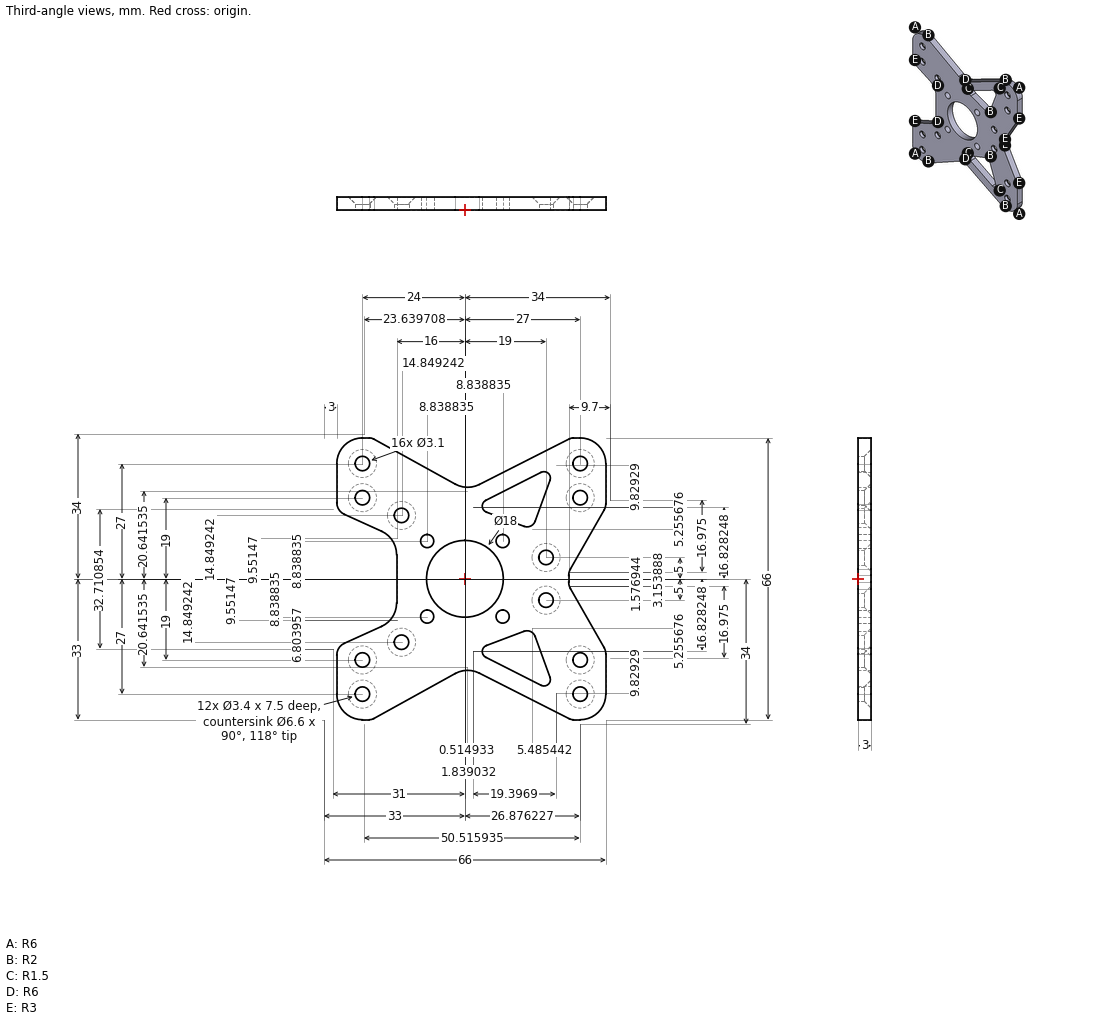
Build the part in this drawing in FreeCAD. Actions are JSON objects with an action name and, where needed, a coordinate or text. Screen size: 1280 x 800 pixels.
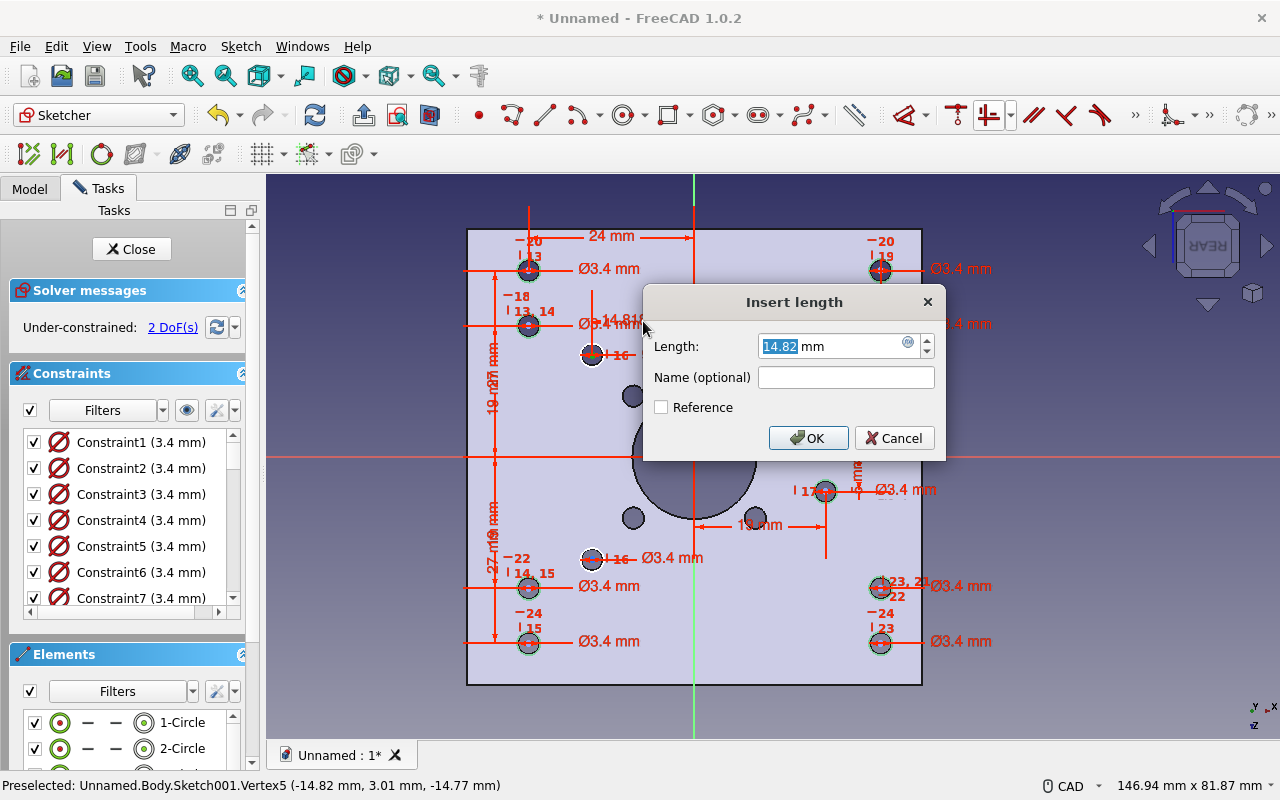
{"action": "type", "text": "14.849242"}
{"action": "key", "text": "Return"}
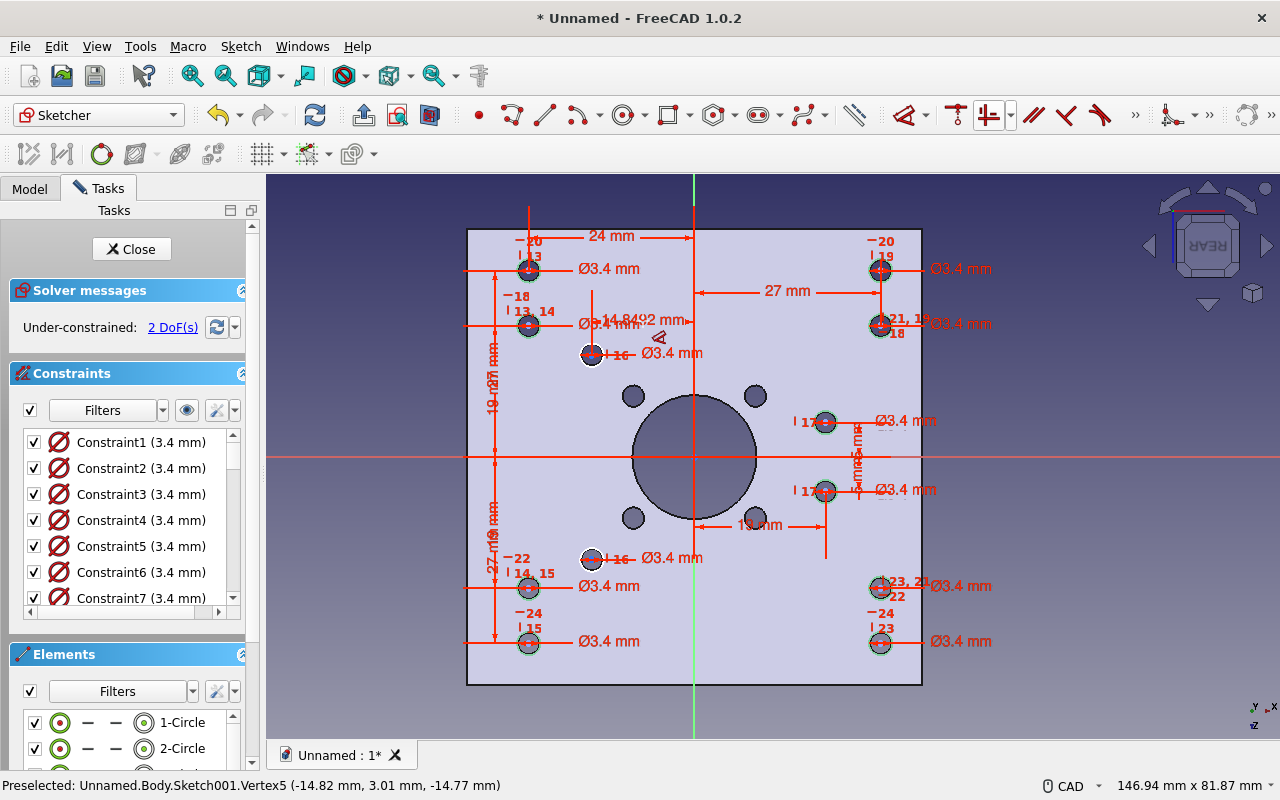
{"action": "left_click", "coordinate": [592, 355]}
{"action": "left_click", "coordinate": [558, 430]}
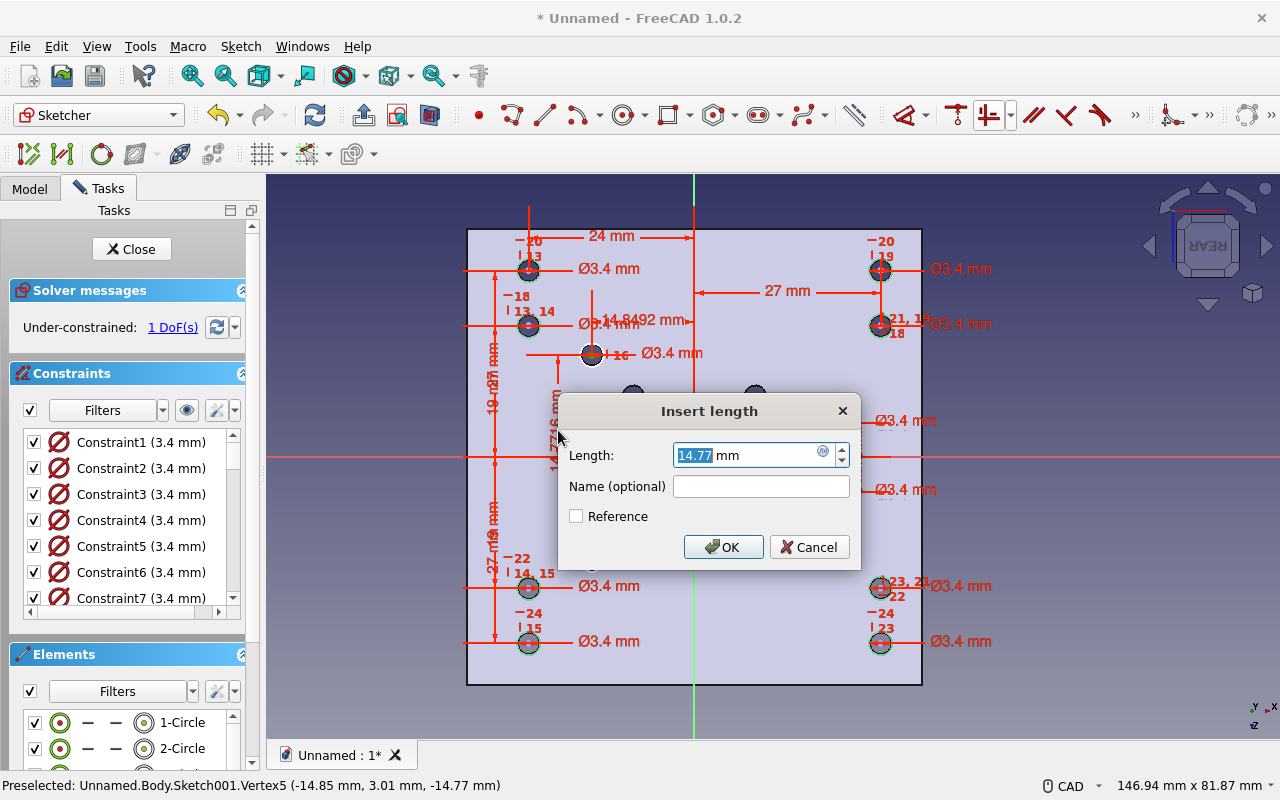
{"action": "type", "text": "14.849242"}
{"action": "key", "text": "Return"}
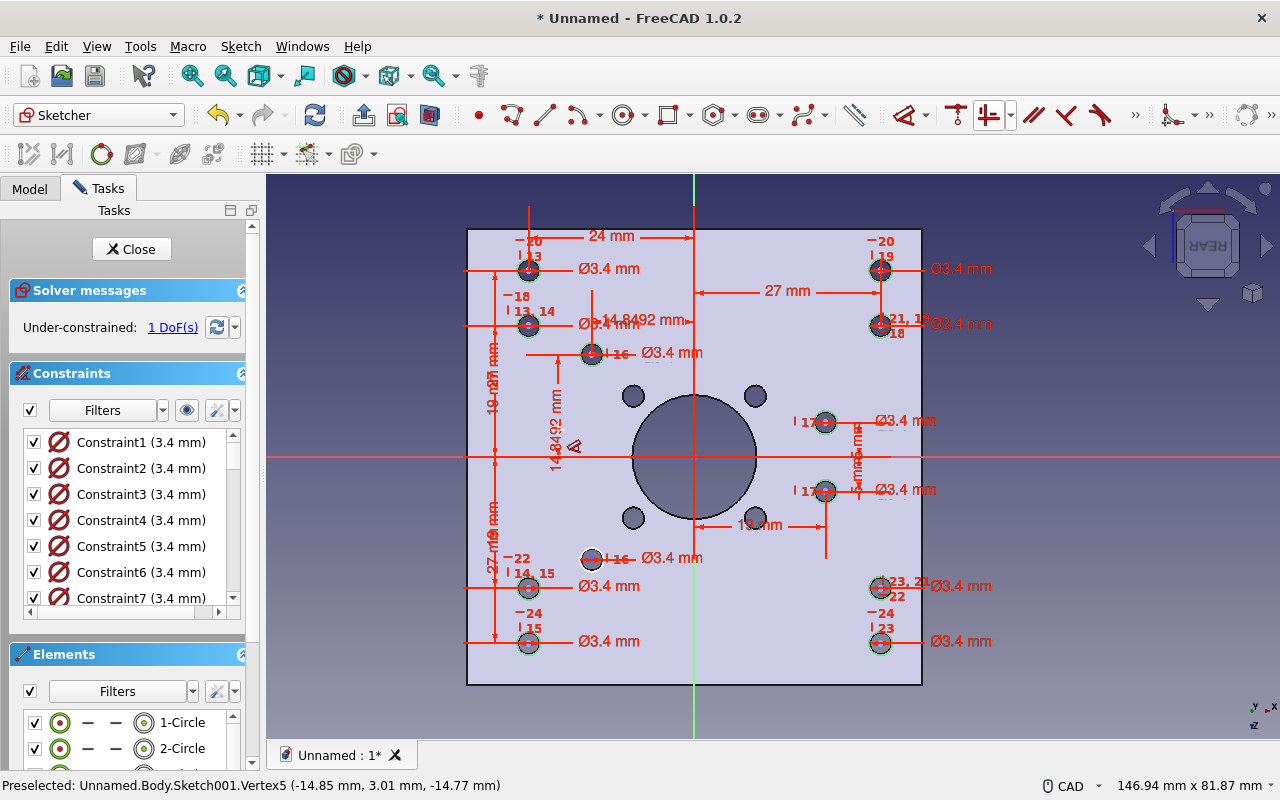
{"action": "left_click", "coordinate": [592, 560]}
{"action": "left_click", "coordinate": [558, 485]}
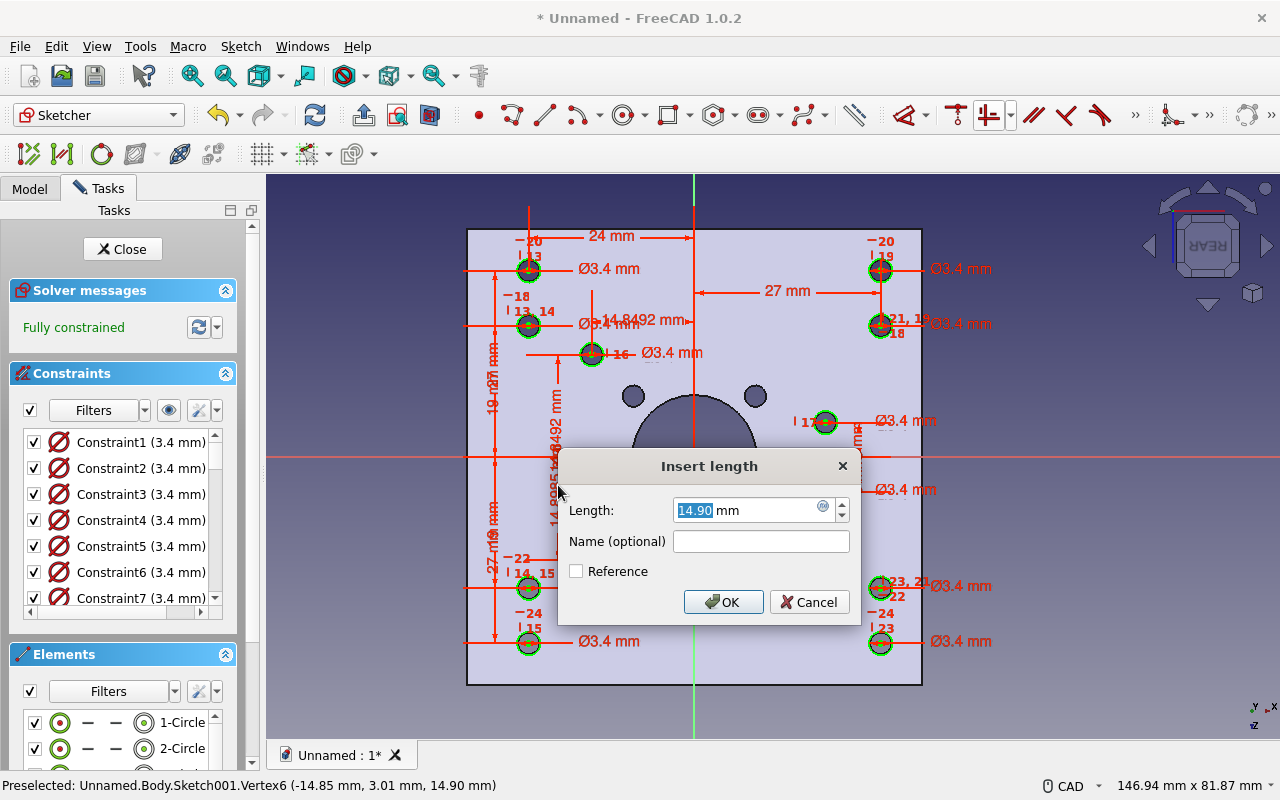
{"action": "type", "text": "14.849242"}
{"action": "key", "text": "Return"}
{"action": "key", "text": "Escape"}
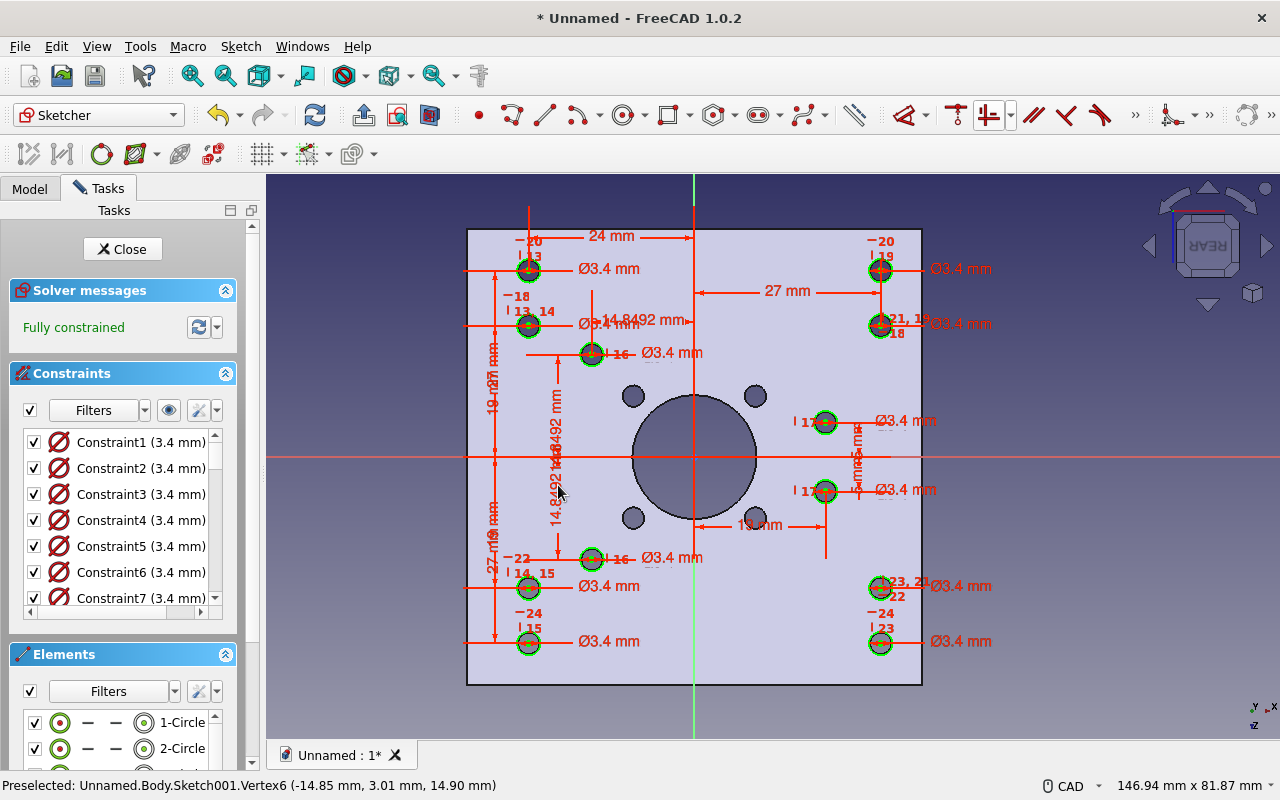
{"action": "left_click", "coordinate": [123, 249]}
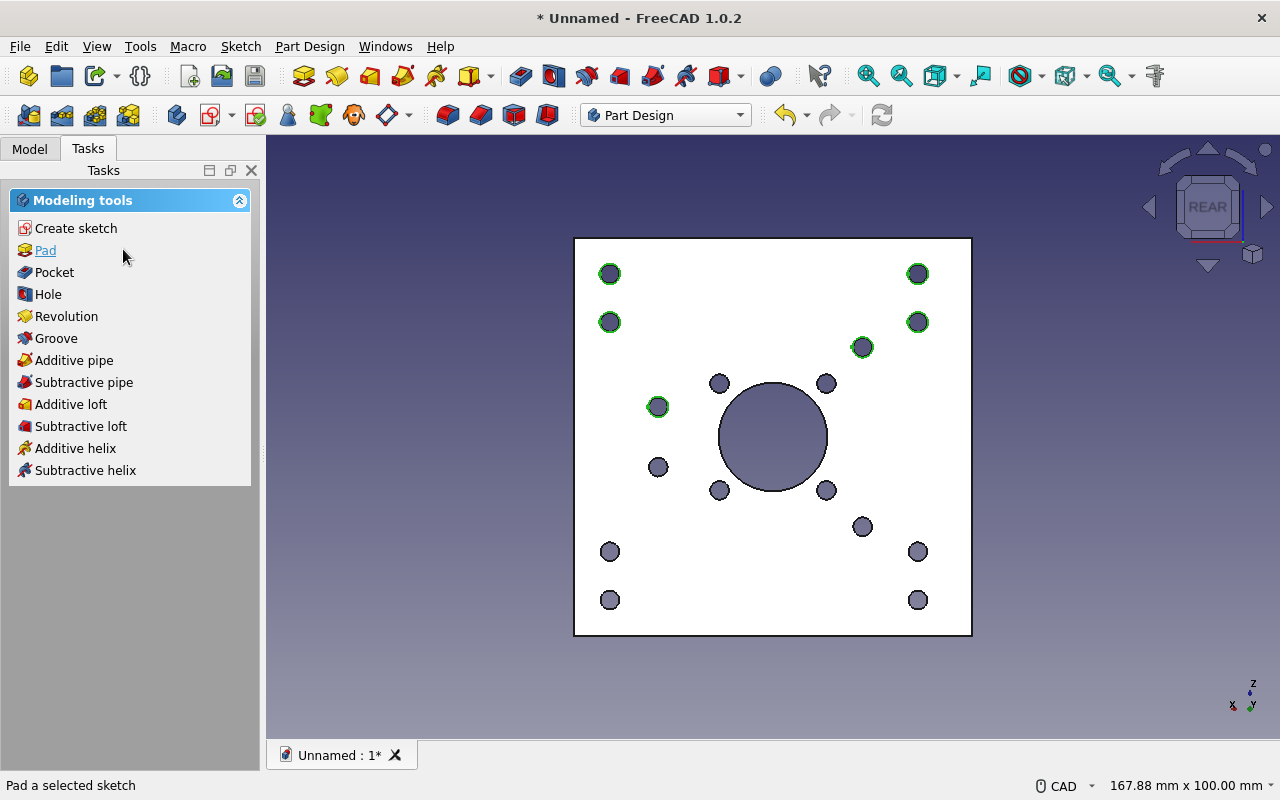
{"action": "left_click", "coordinate": [554, 76]}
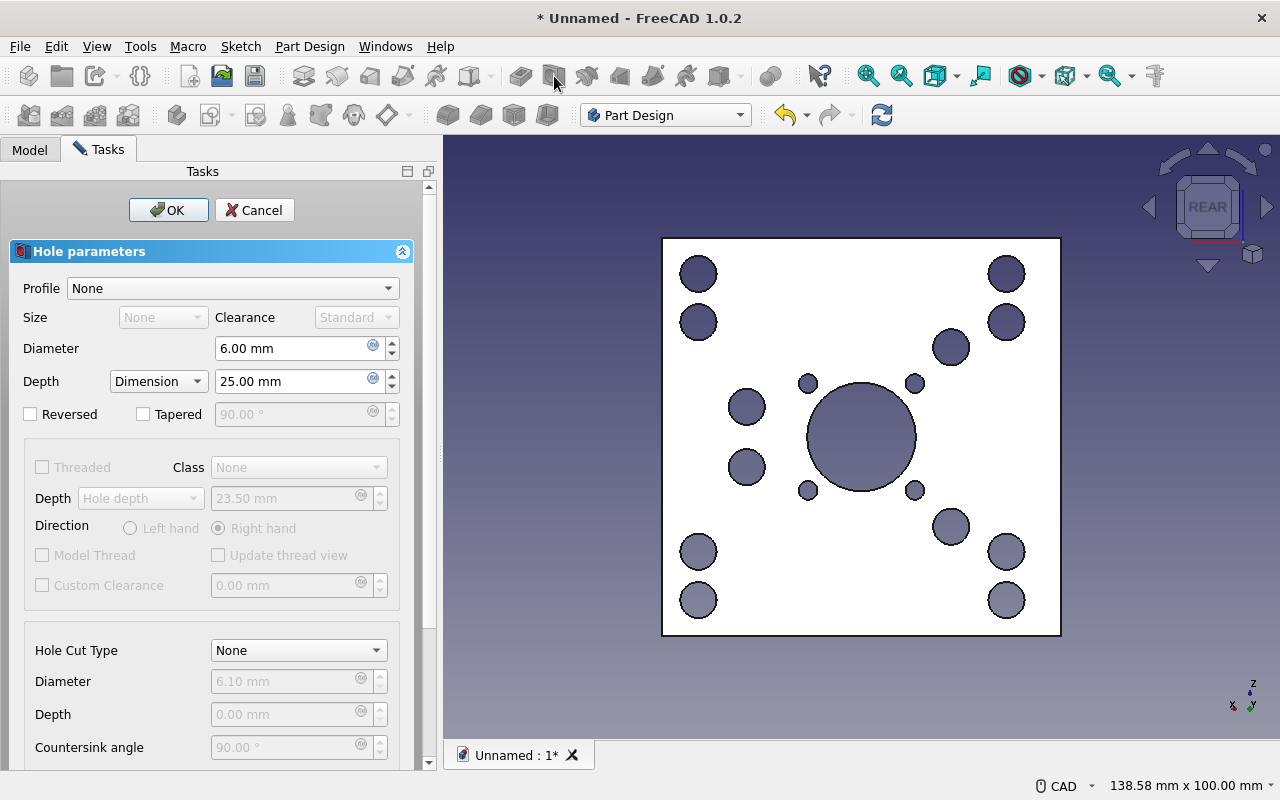
{"action": "triple_click", "coordinate": [300, 348]}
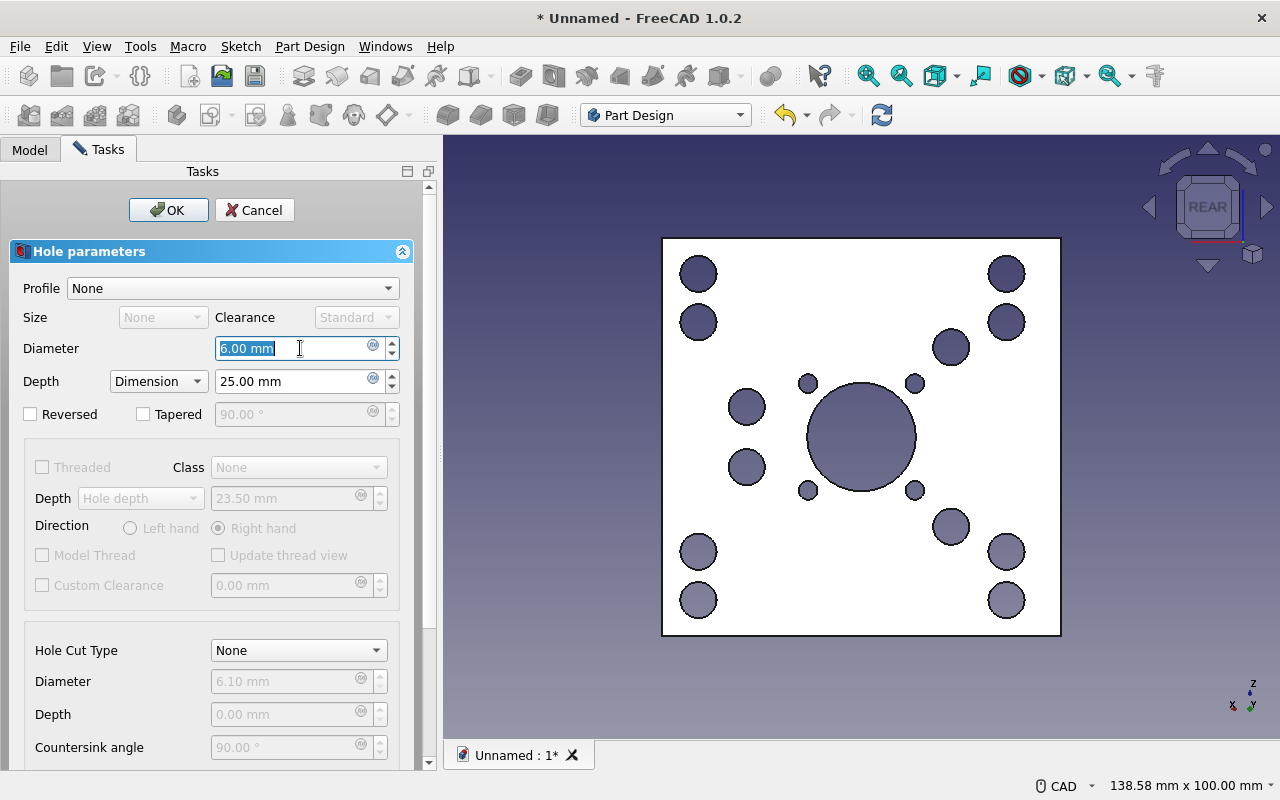
{"action": "type", "text": "3.4"}
{"action": "key", "text": "Tab"}